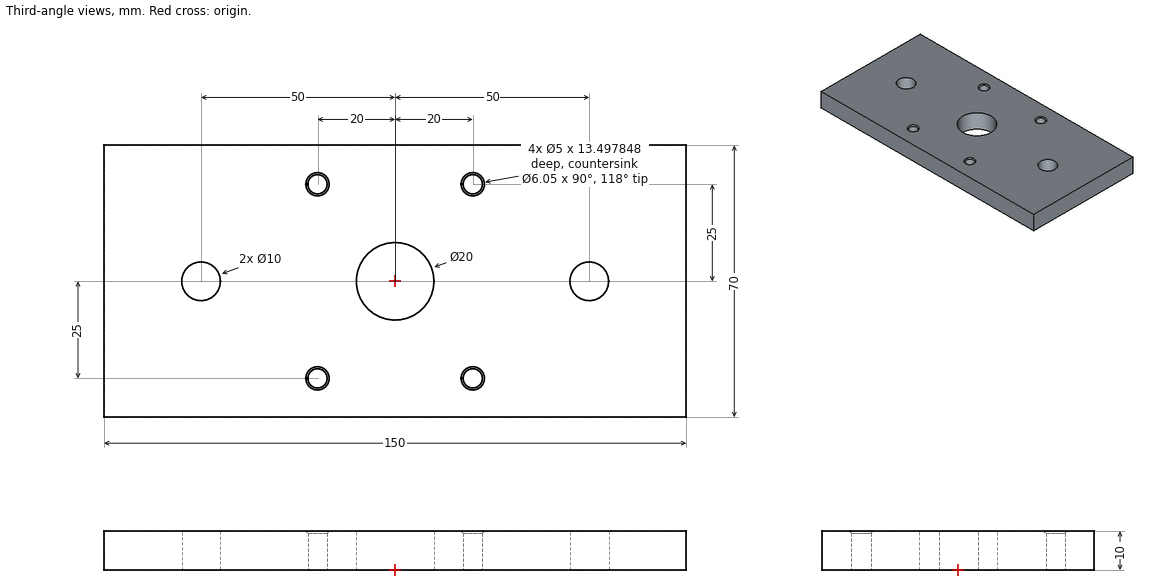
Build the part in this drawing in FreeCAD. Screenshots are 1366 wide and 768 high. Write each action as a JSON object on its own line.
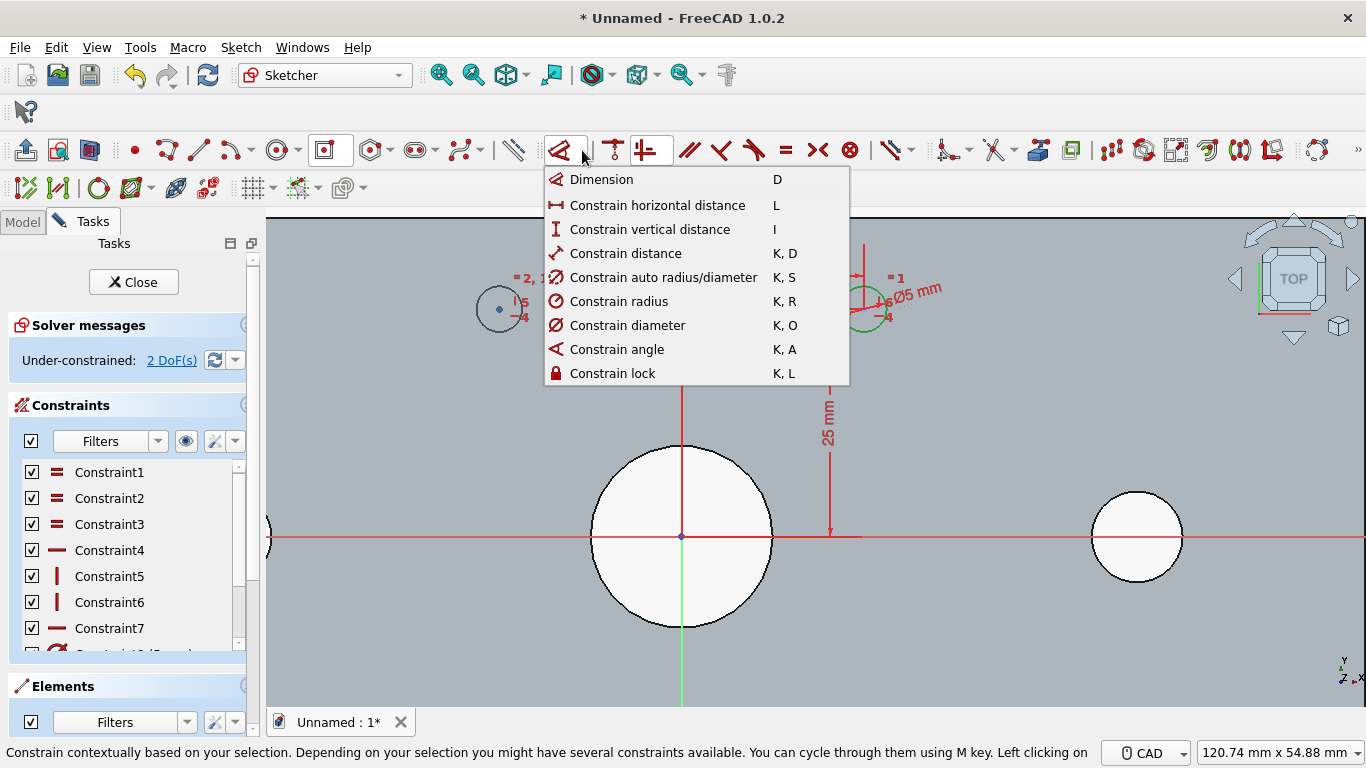
{"action": "left_click", "coordinate": [697, 205]}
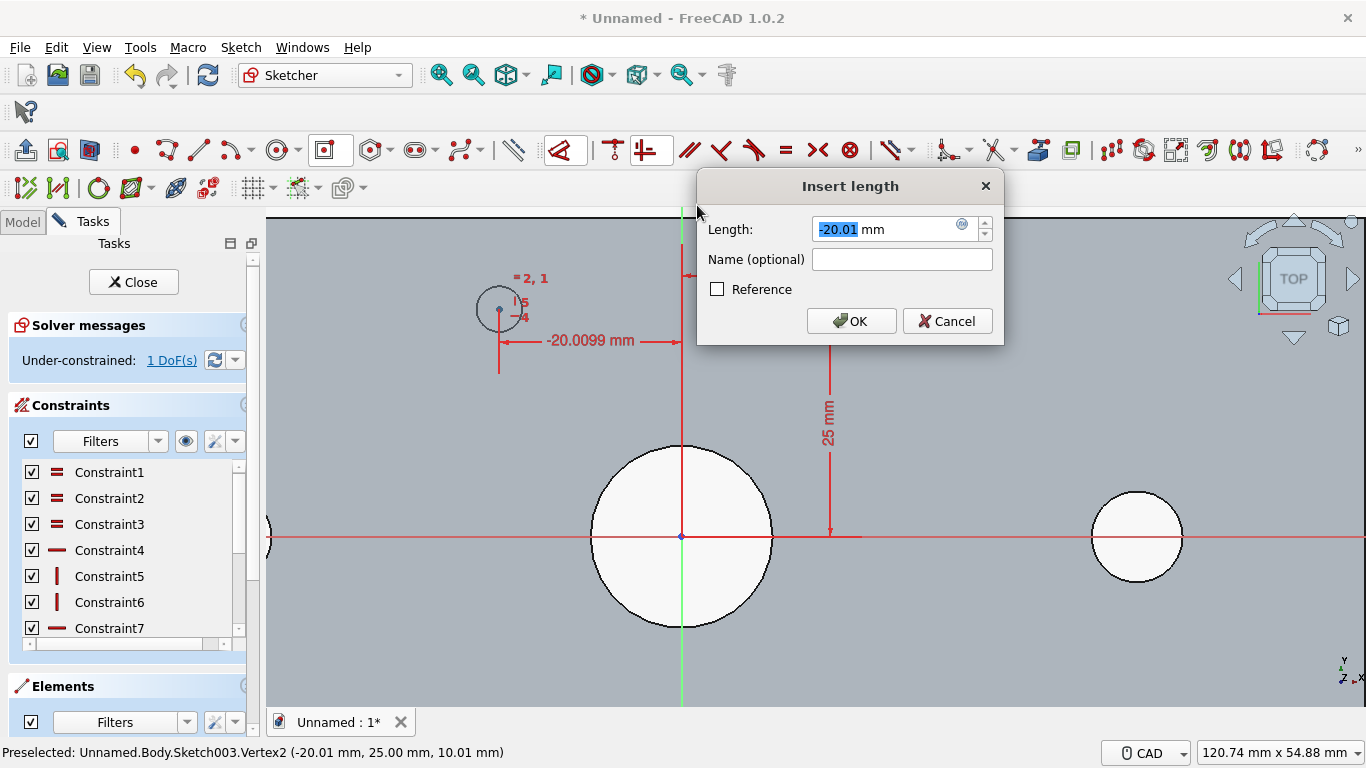
{"action": "type", "text": "-20"}
{"action": "key", "text": "Return"}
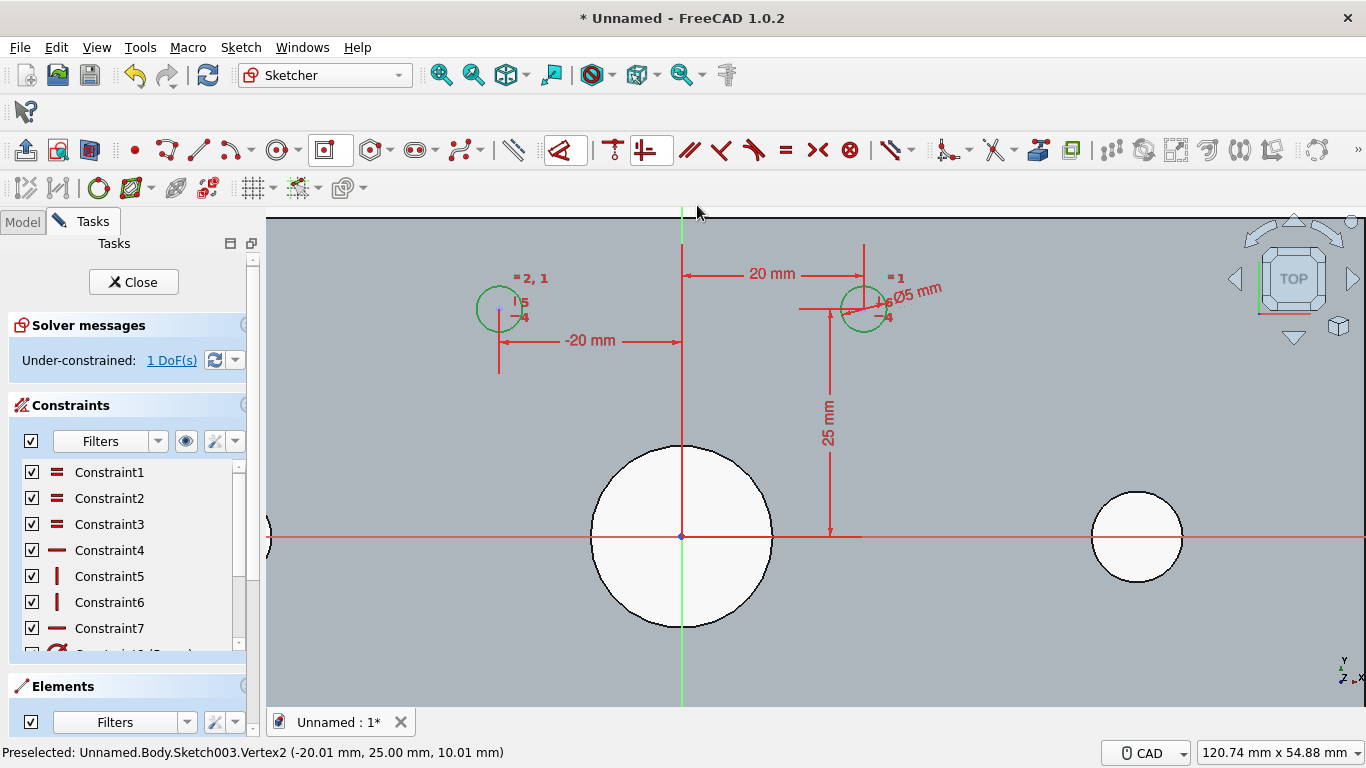
{"action": "scroll", "coordinate": [881, 295], "scroll_direction": "down", "scroll_amount": 2}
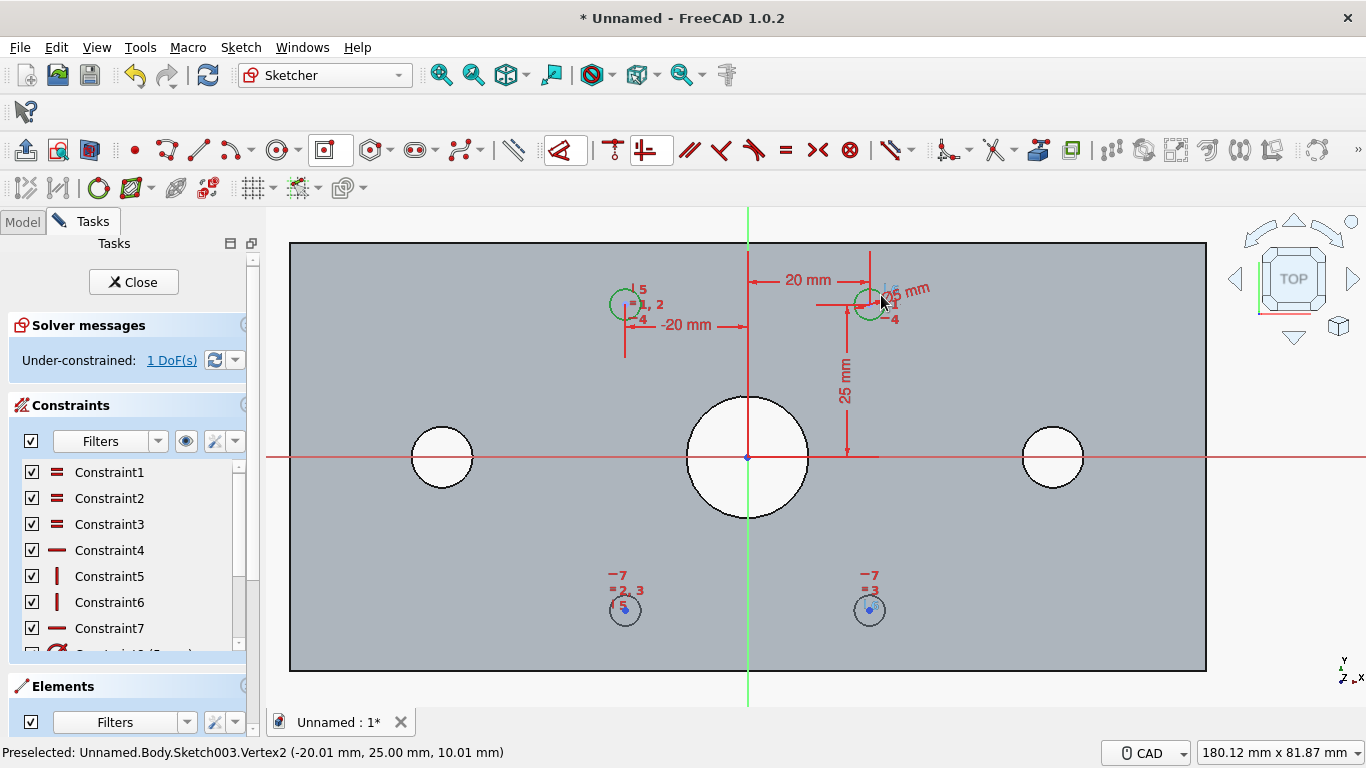
{"action": "left_click", "coordinate": [625, 611]}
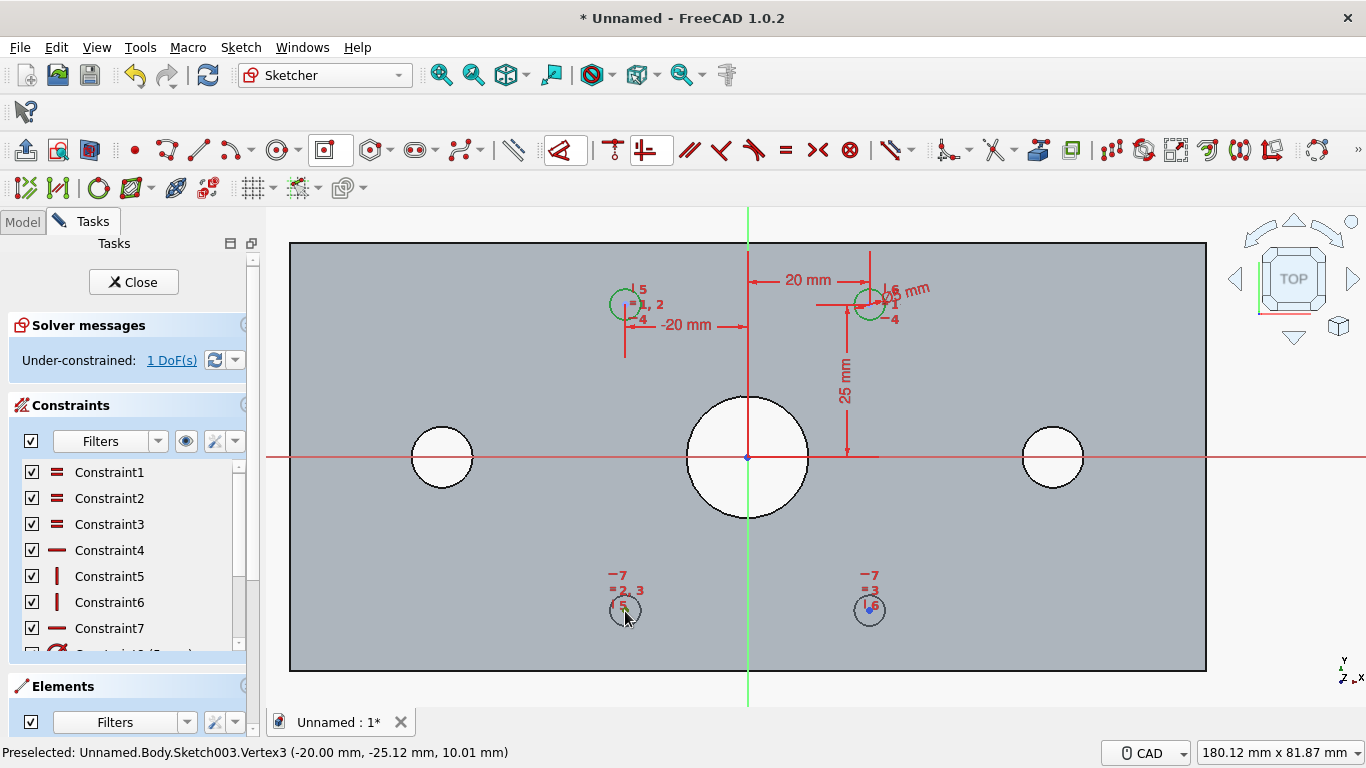
{"action": "left_click", "coordinate": [582, 150]}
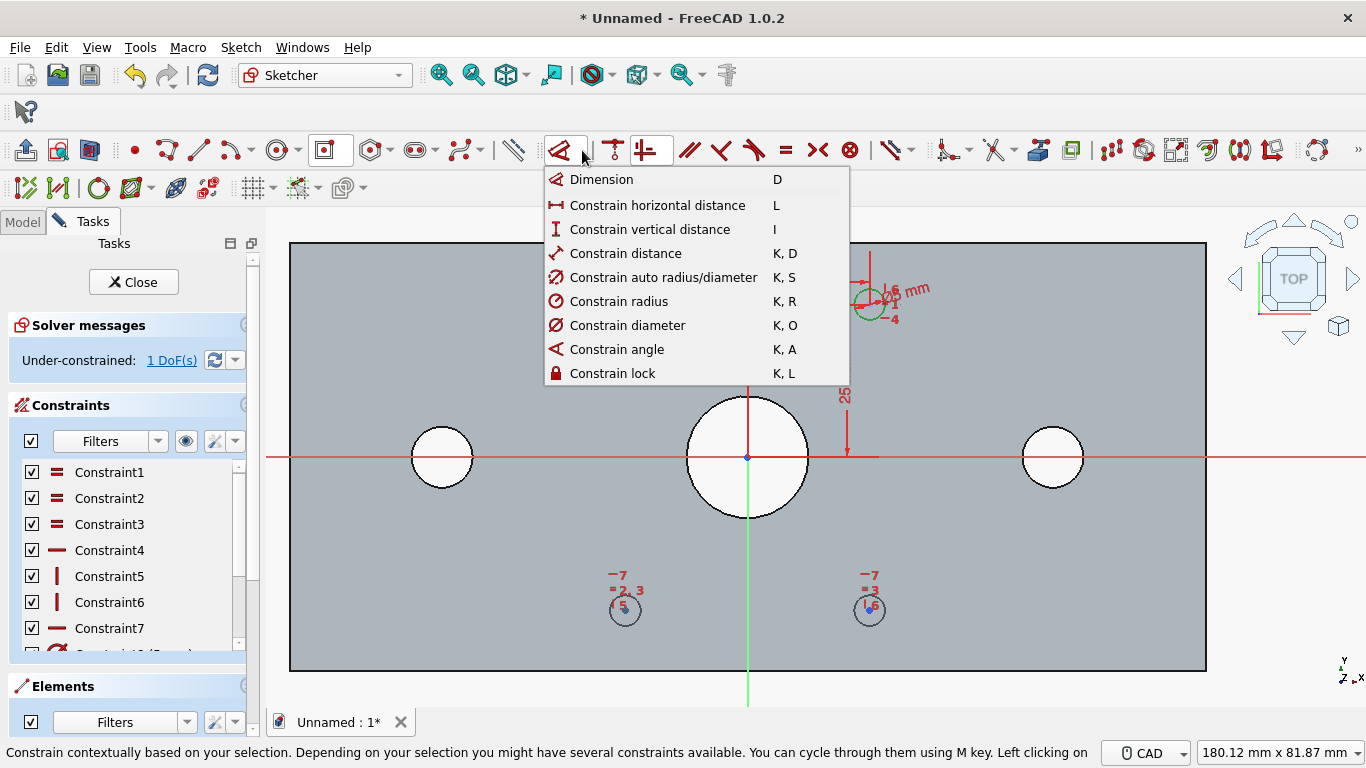
{"action": "left_click", "coordinate": [697, 229]}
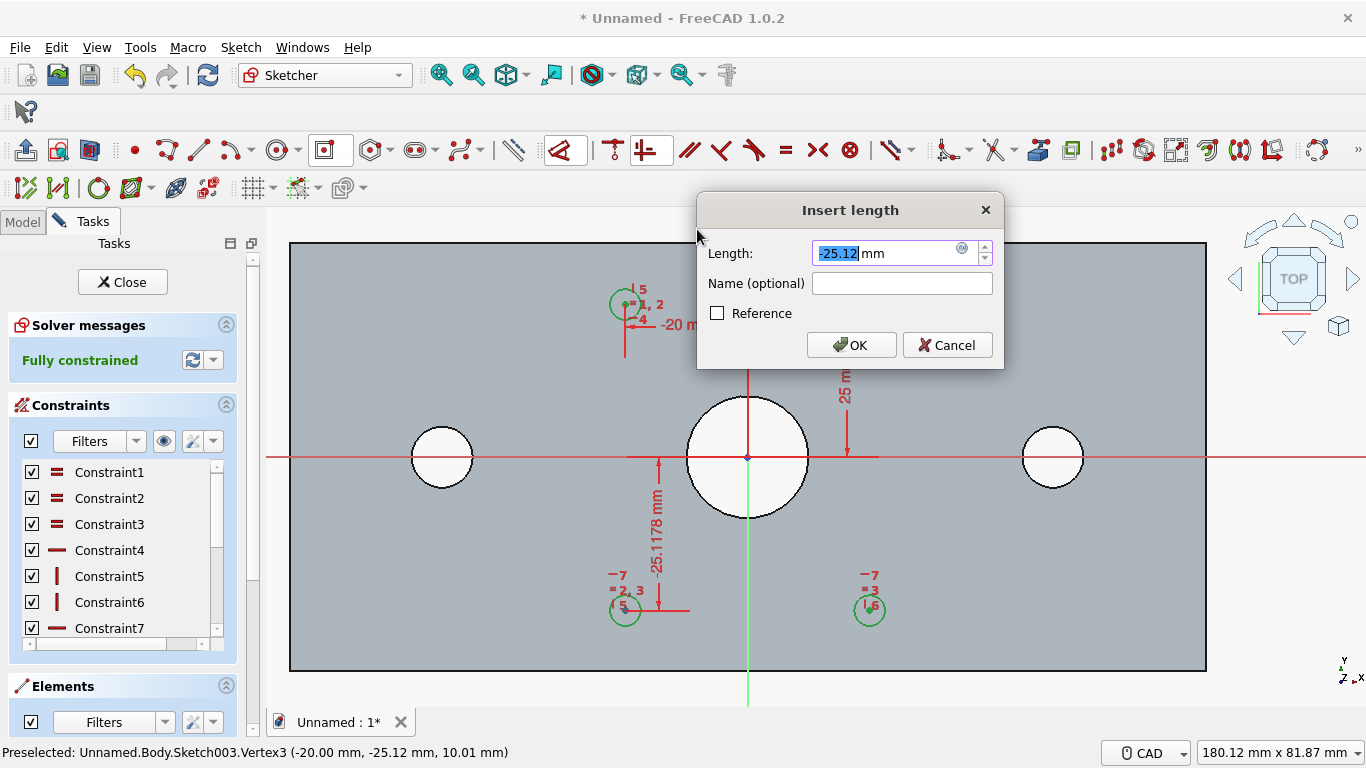
{"action": "type", "text": "-25"}
{"action": "key", "text": "Return"}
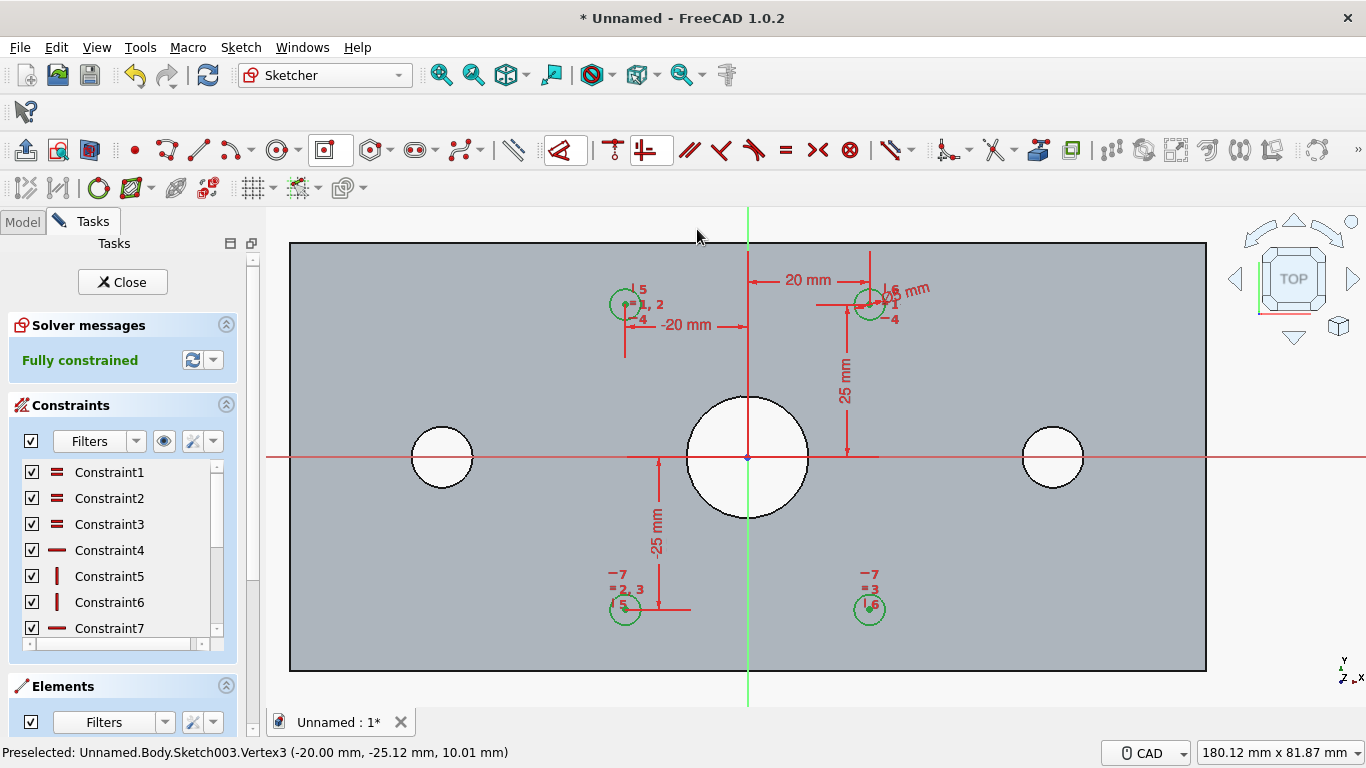
{"action": "left_click", "coordinate": [123, 282]}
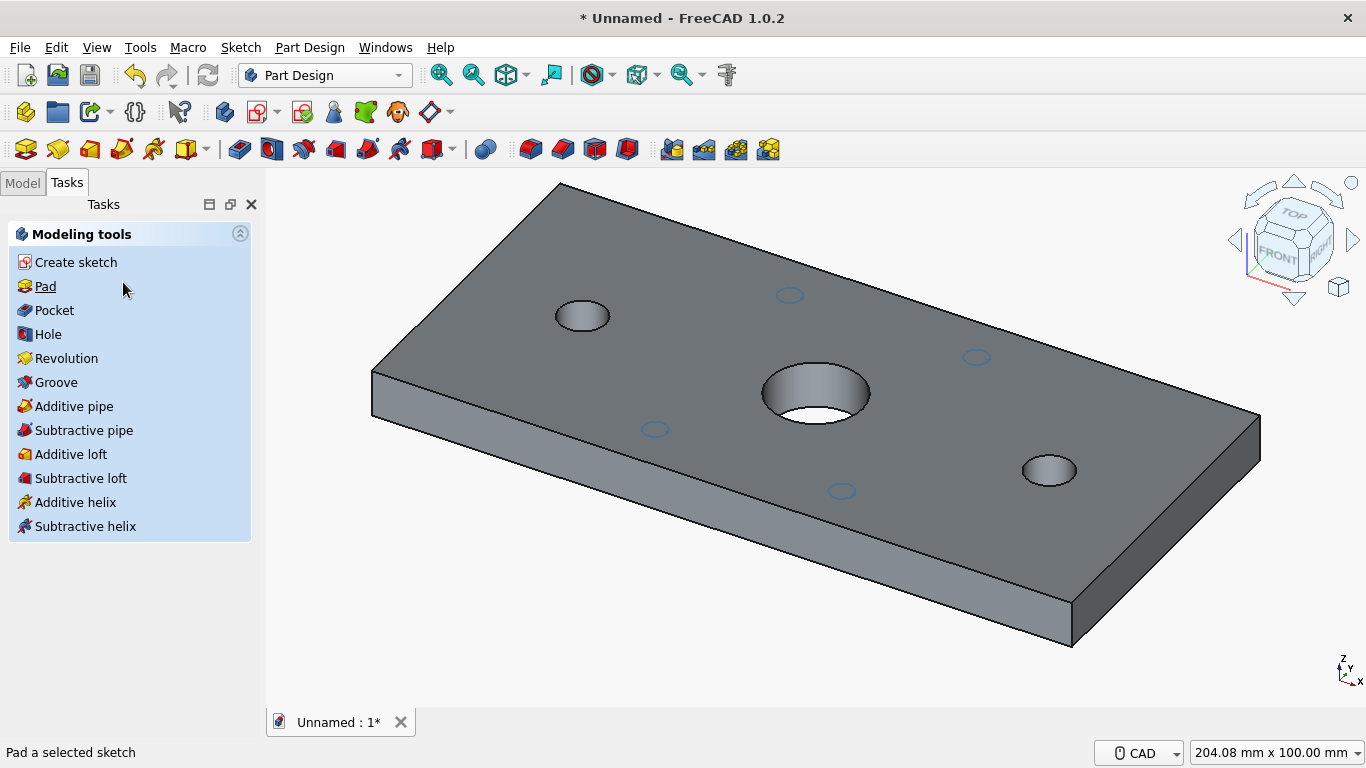
{"action": "left_click", "coordinate": [272, 150]}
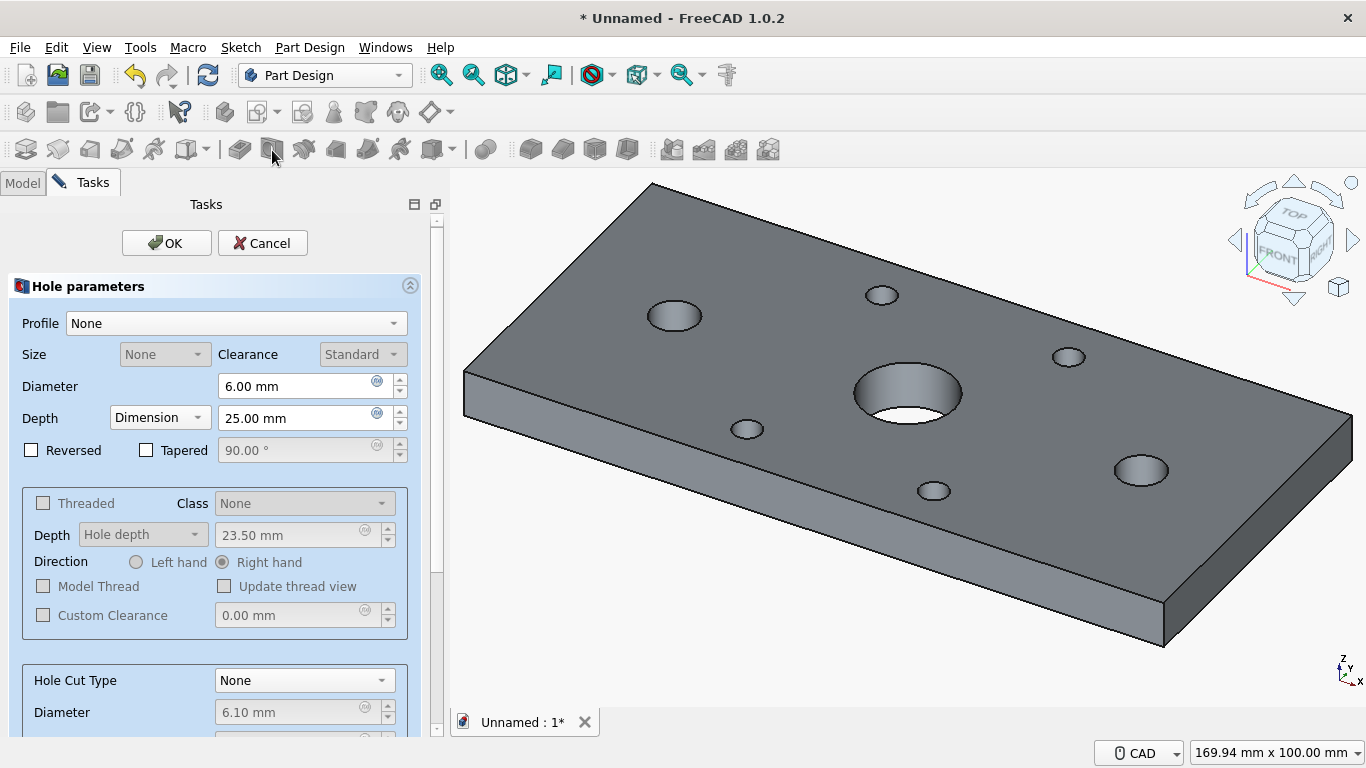
{"action": "triple_click", "coordinate": [305, 386]}